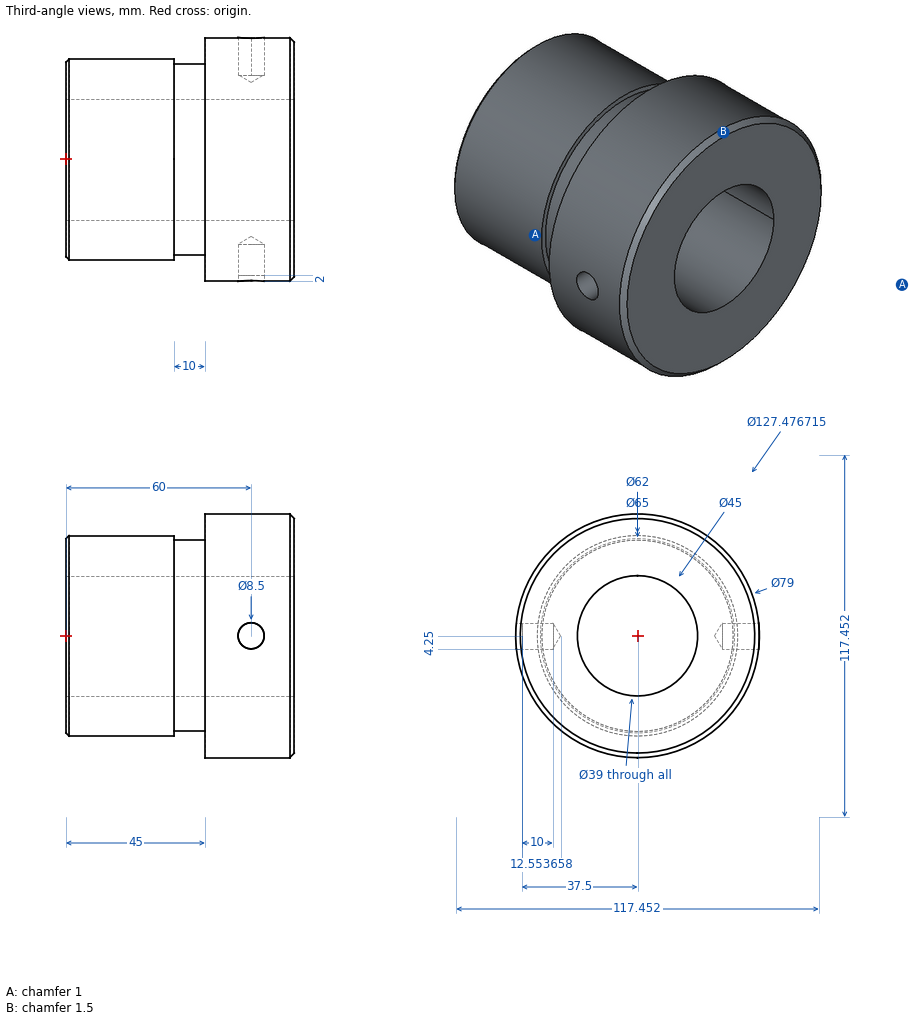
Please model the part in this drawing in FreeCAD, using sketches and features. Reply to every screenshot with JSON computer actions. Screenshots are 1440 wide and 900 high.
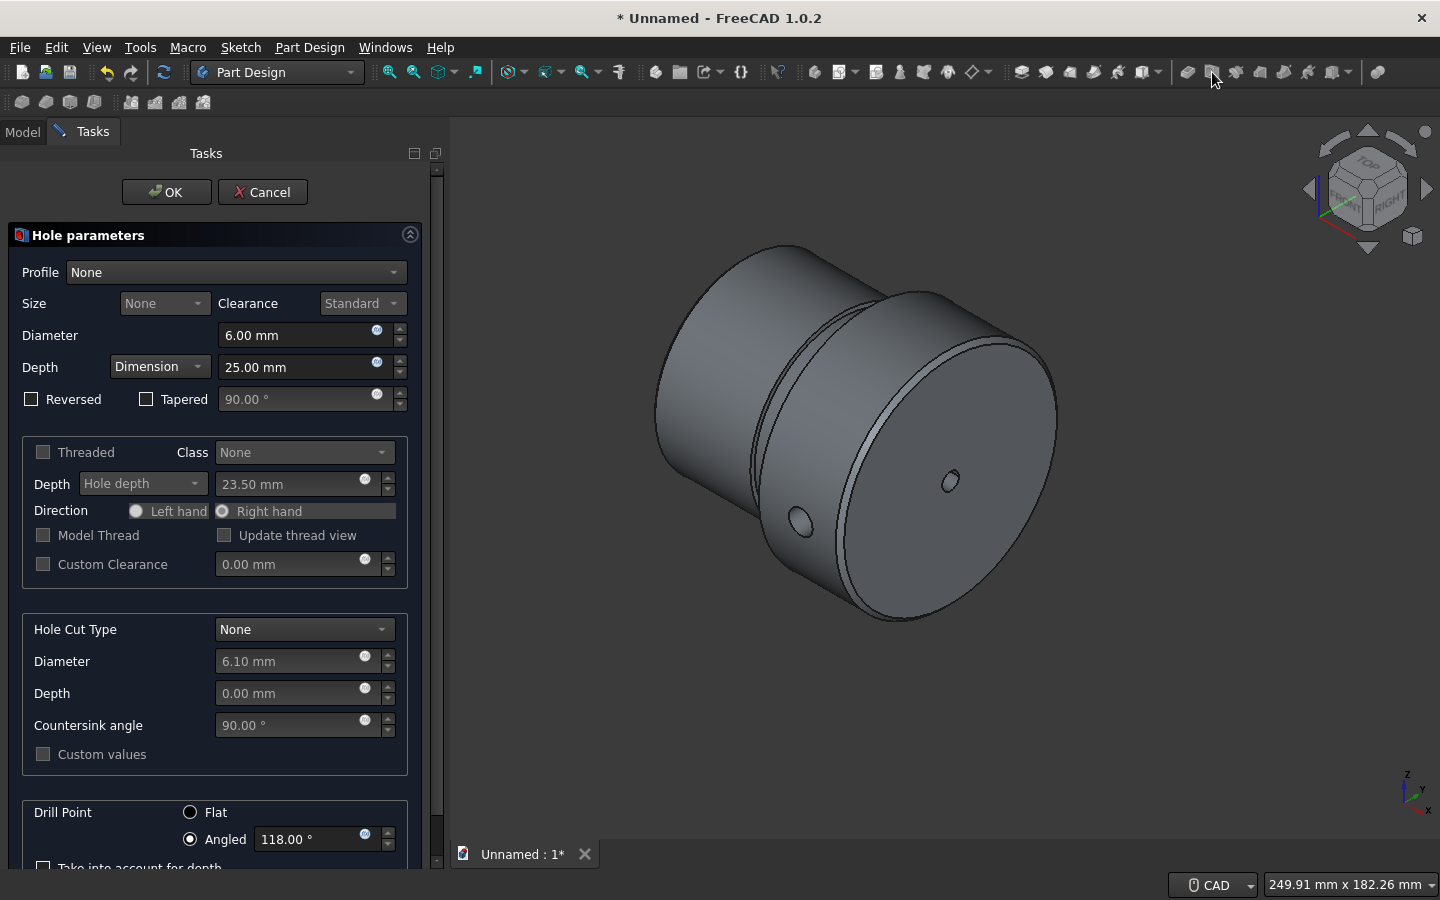
{"action": "triple_click", "coordinate": [305, 335]}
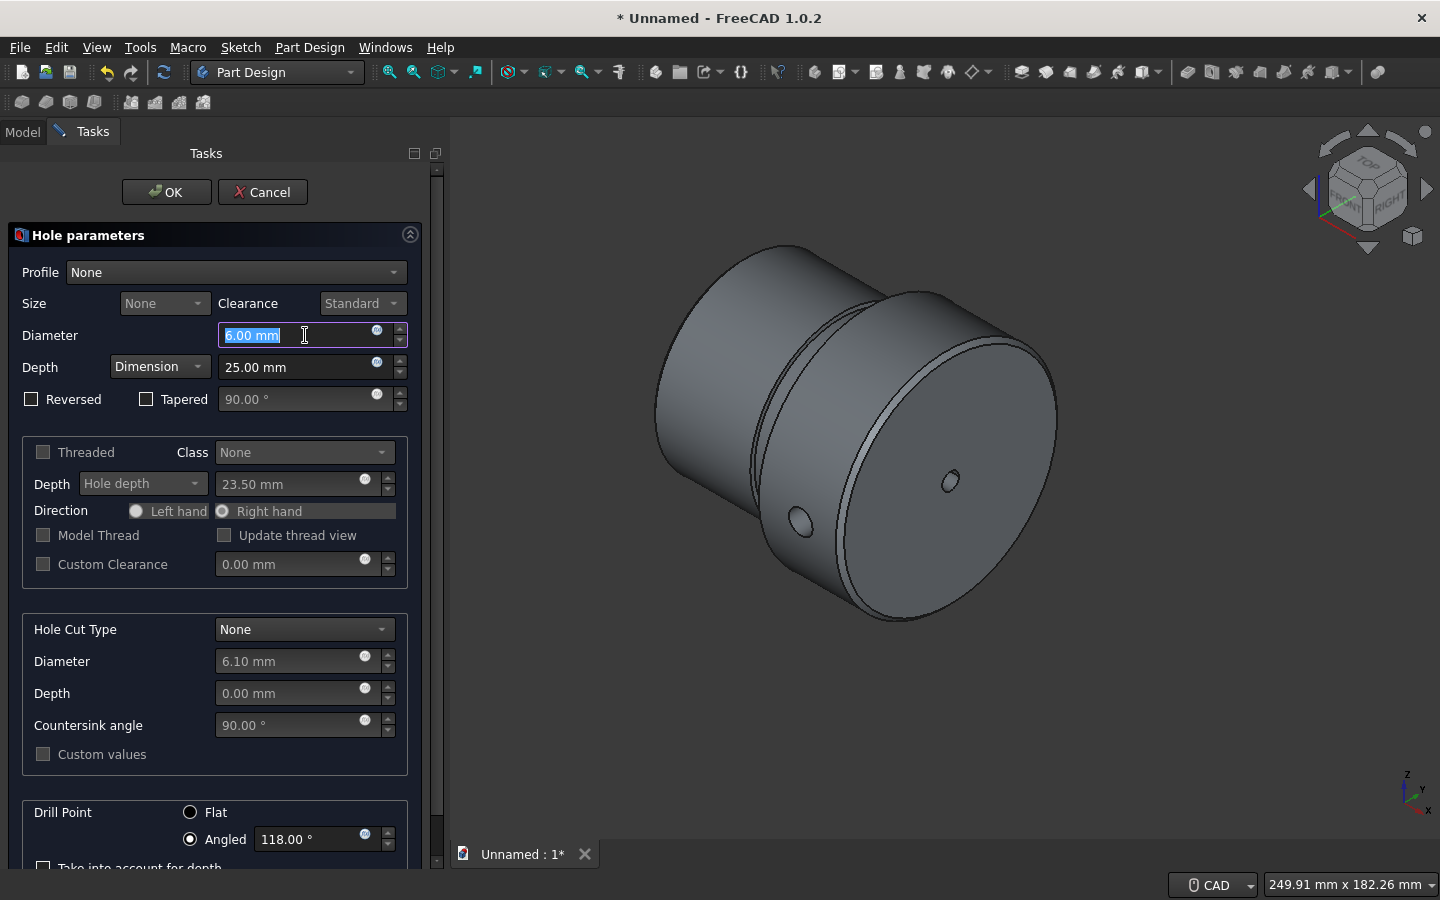
{"action": "type", "text": "39"}
{"action": "key", "text": "Tab"}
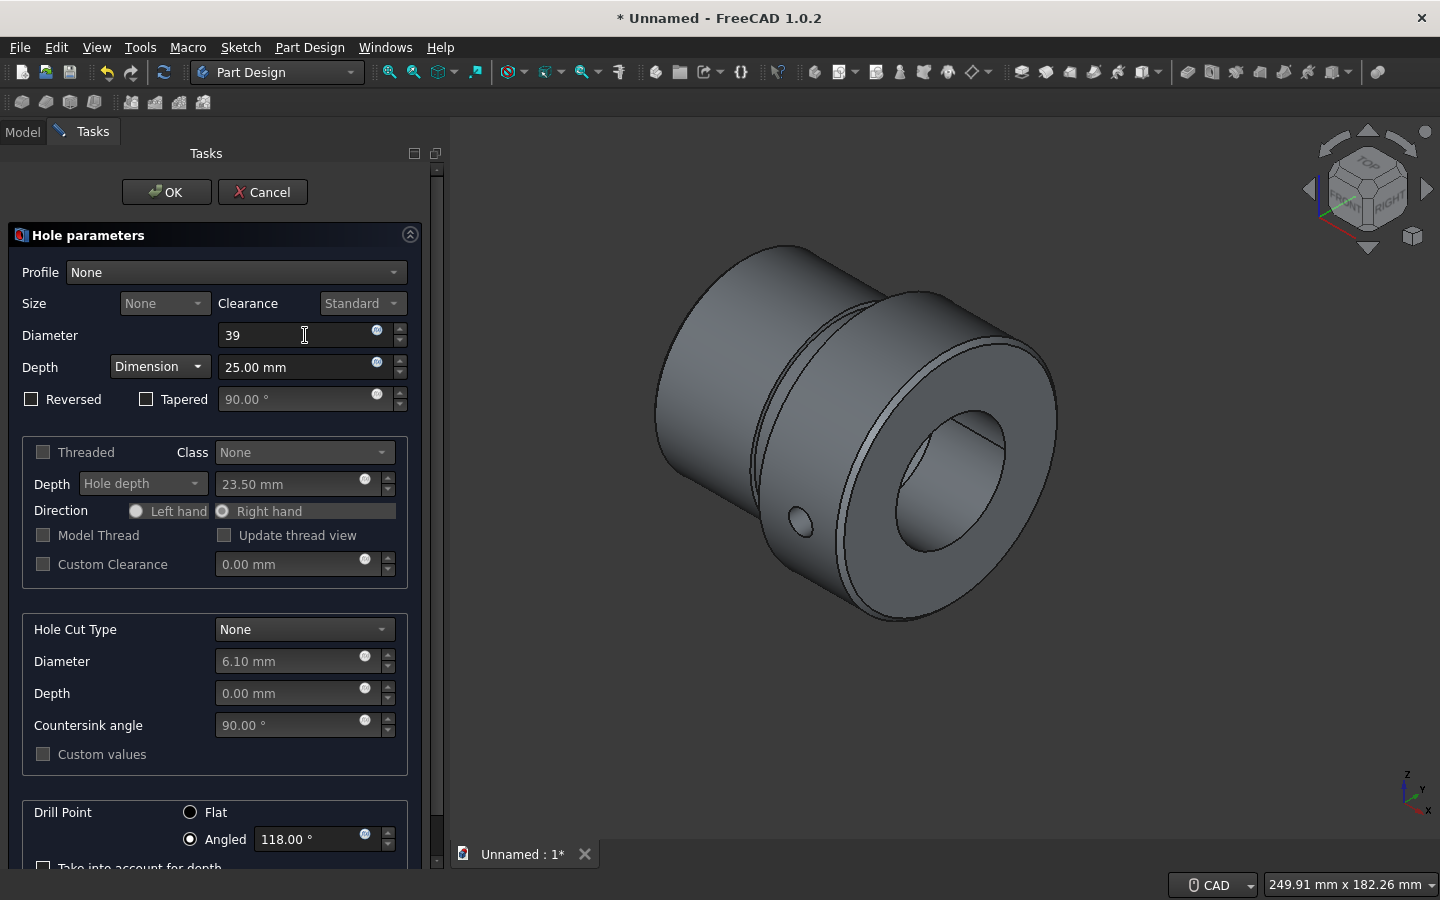
{"action": "left_click", "coordinate": [161, 366]}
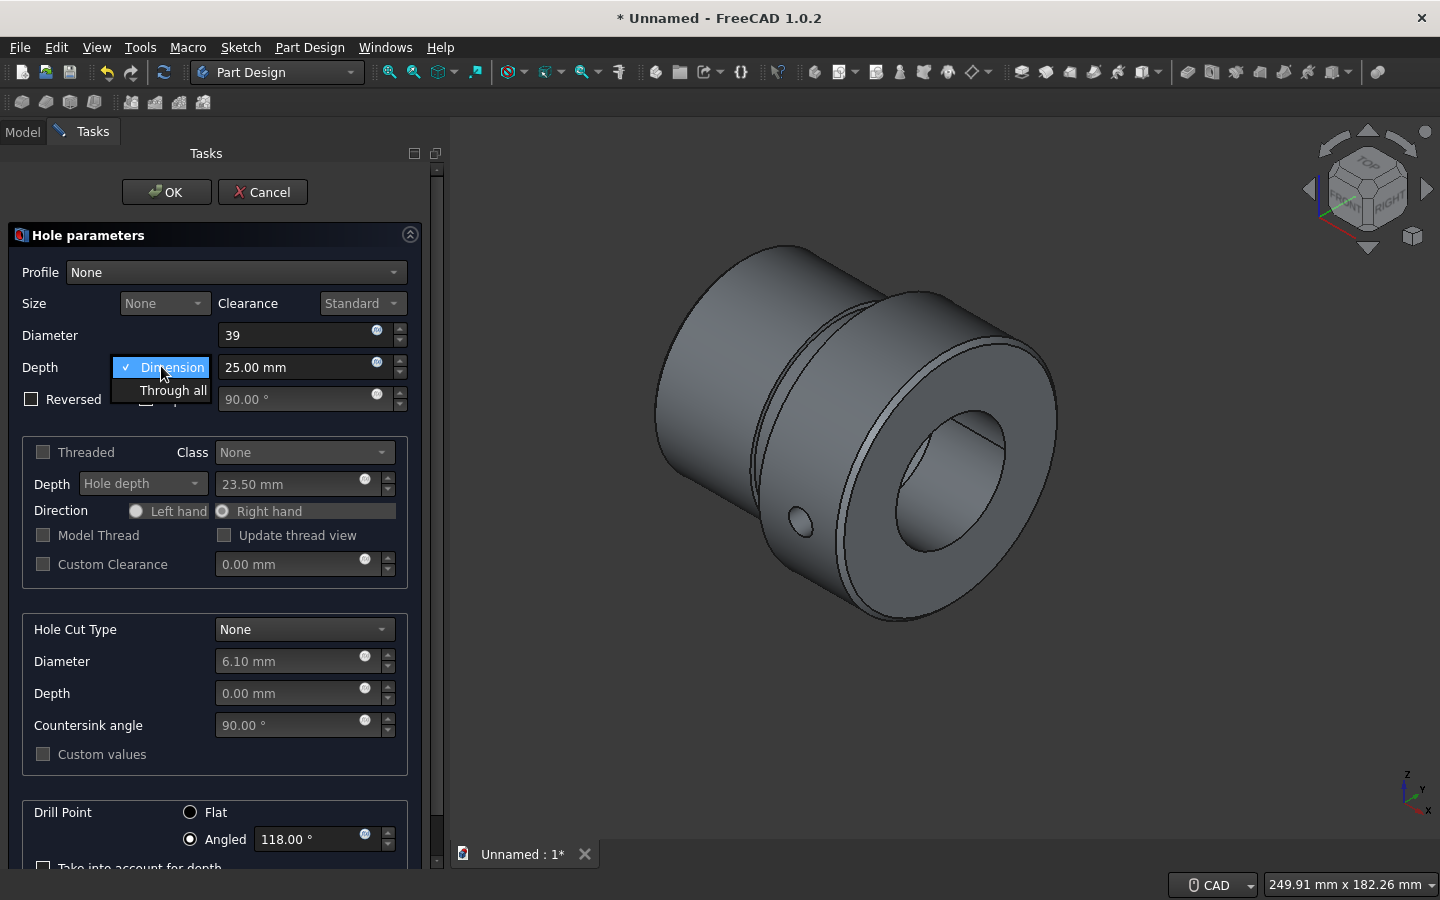
{"action": "left_click", "coordinate": [160, 390]}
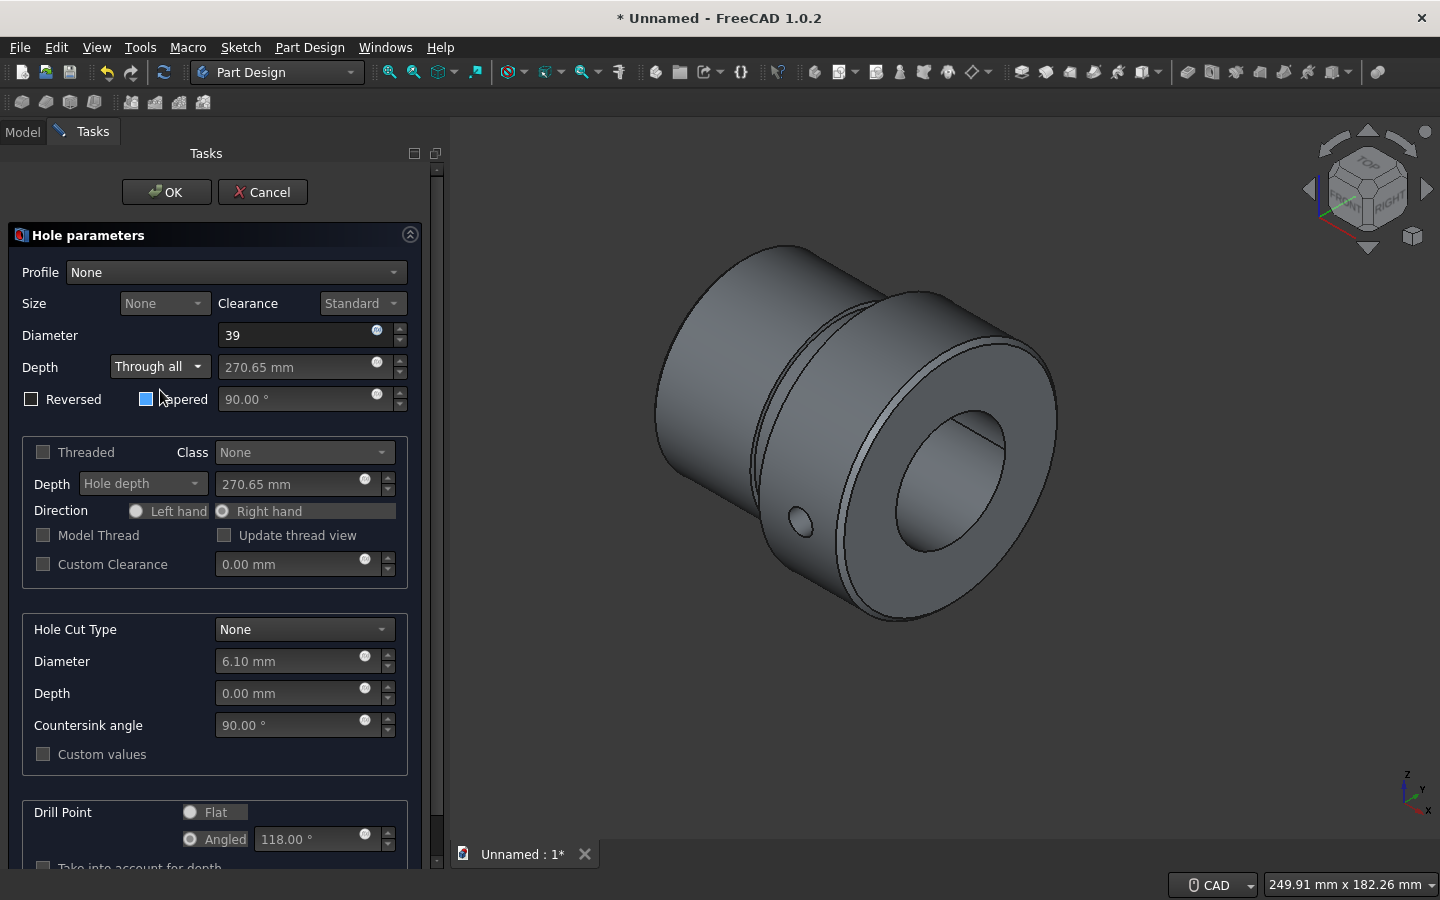
{"action": "left_click", "coordinate": [167, 192]}